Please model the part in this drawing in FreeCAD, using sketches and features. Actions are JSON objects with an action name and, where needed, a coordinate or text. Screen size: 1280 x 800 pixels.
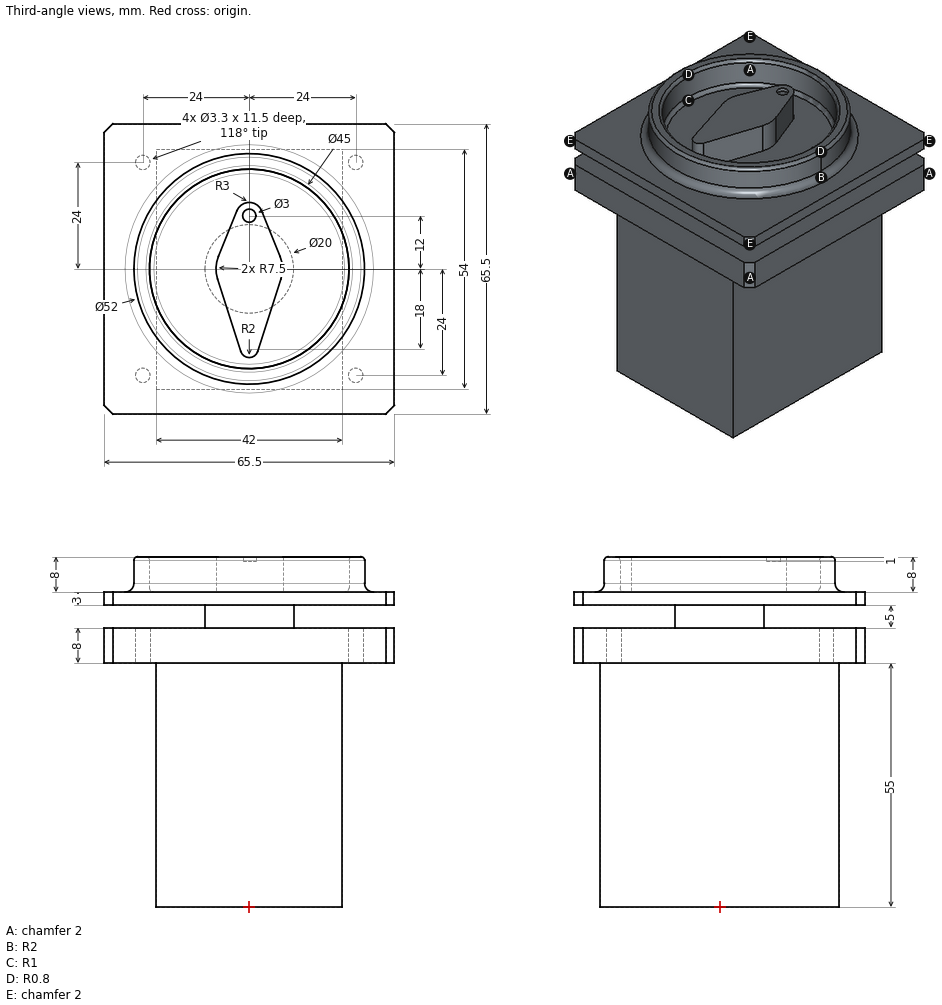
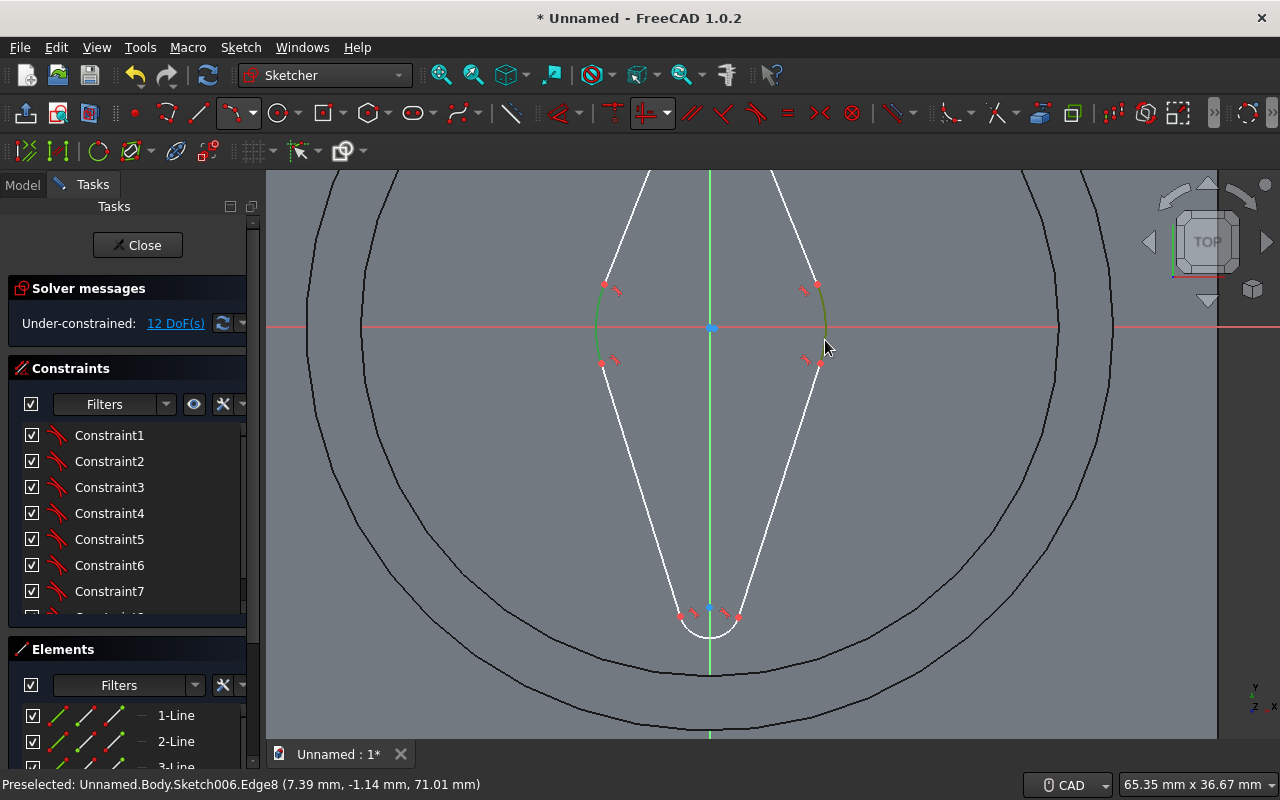
{"action": "left_click", "coordinate": [614, 114]}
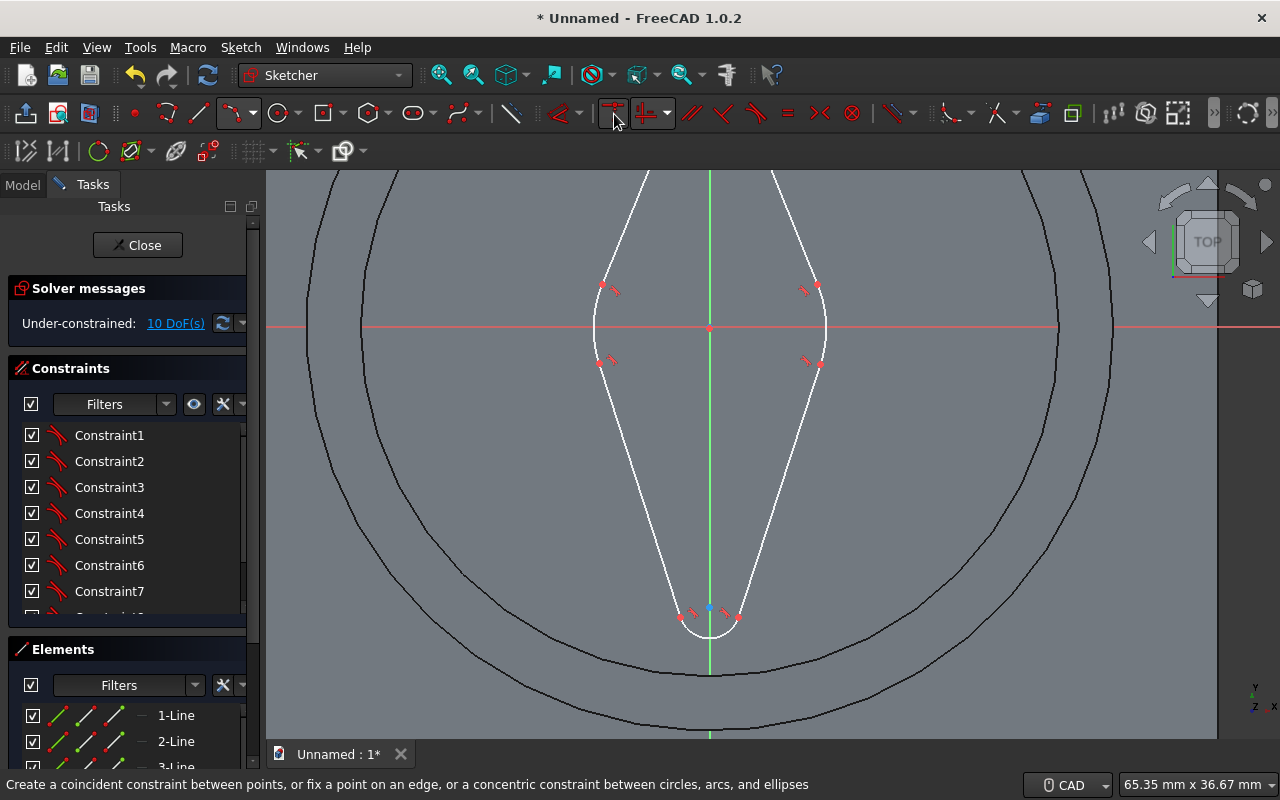
{"action": "scroll", "coordinate": [710, 328], "scroll_direction": "up", "scroll_amount": 2}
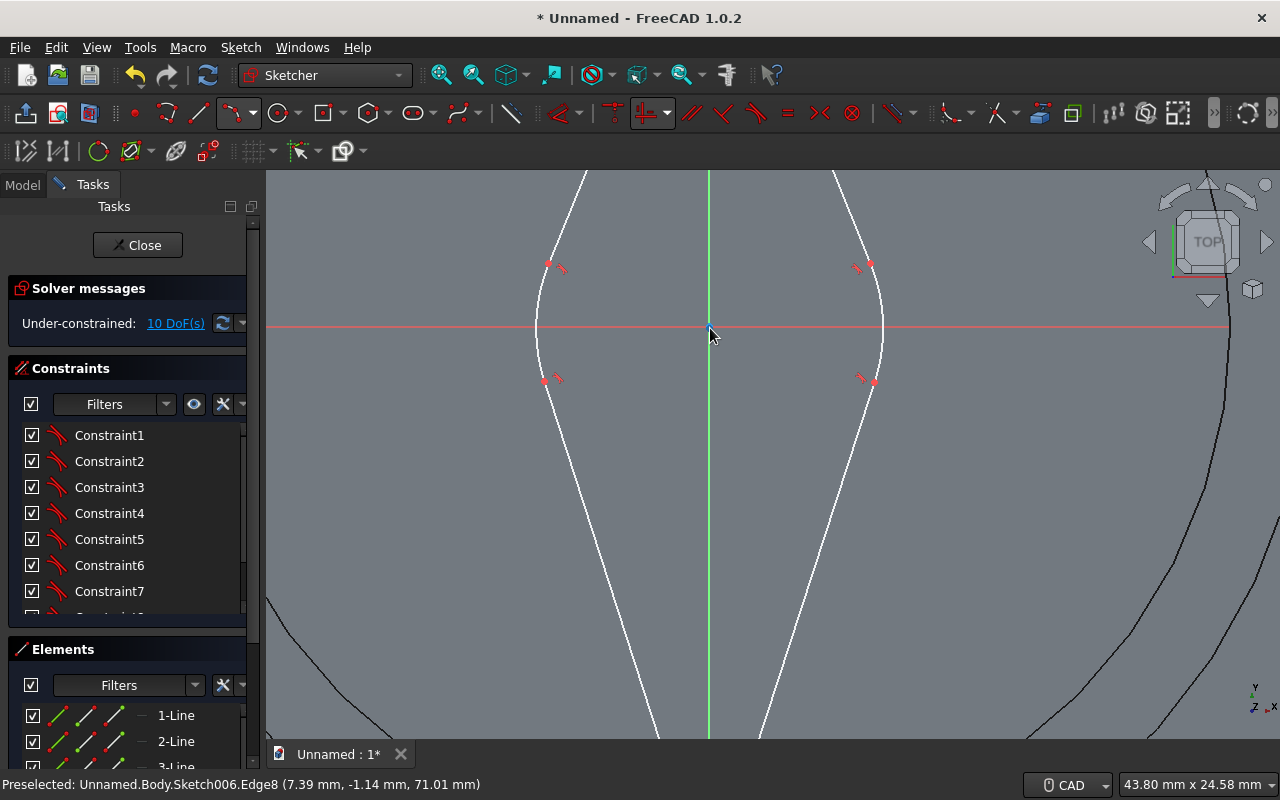
{"action": "left_click_drag", "start_coordinate": [699, 317], "coordinate": [719, 339]}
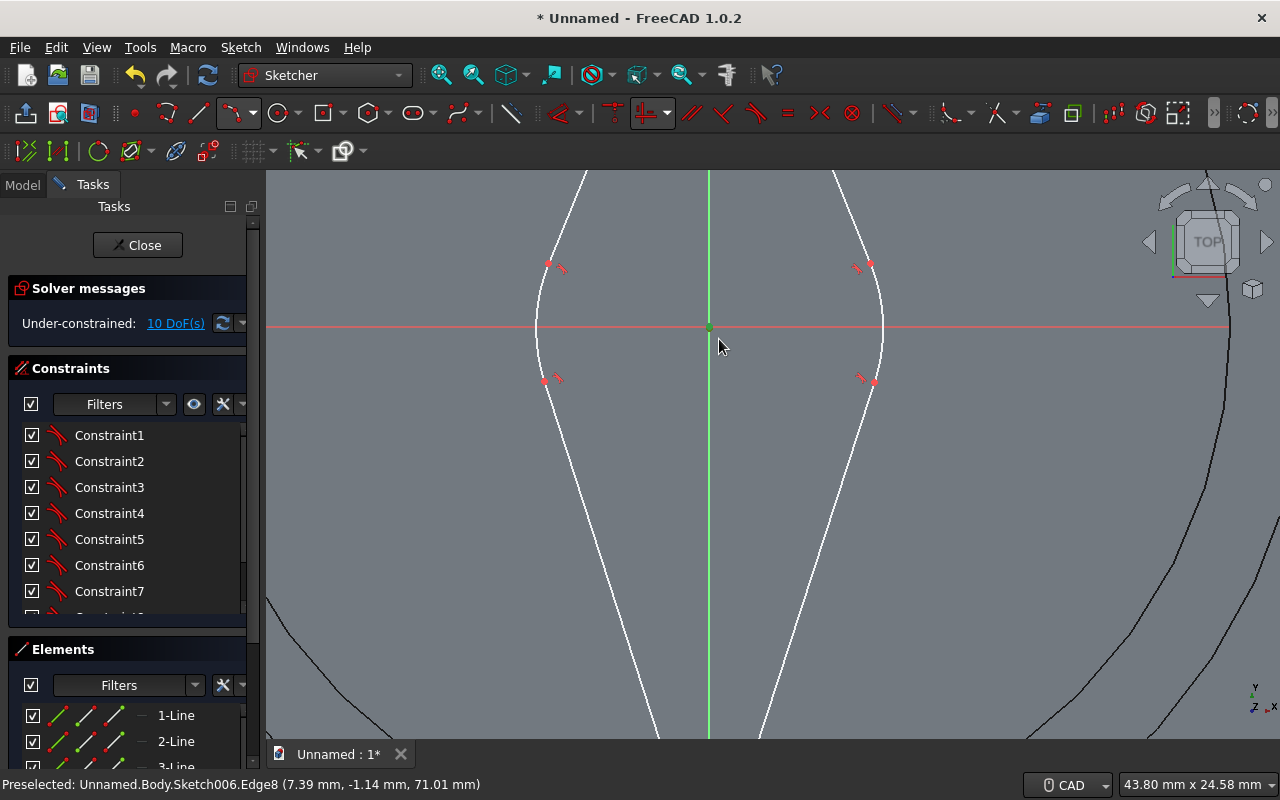
{"action": "left_click", "coordinate": [614, 114]}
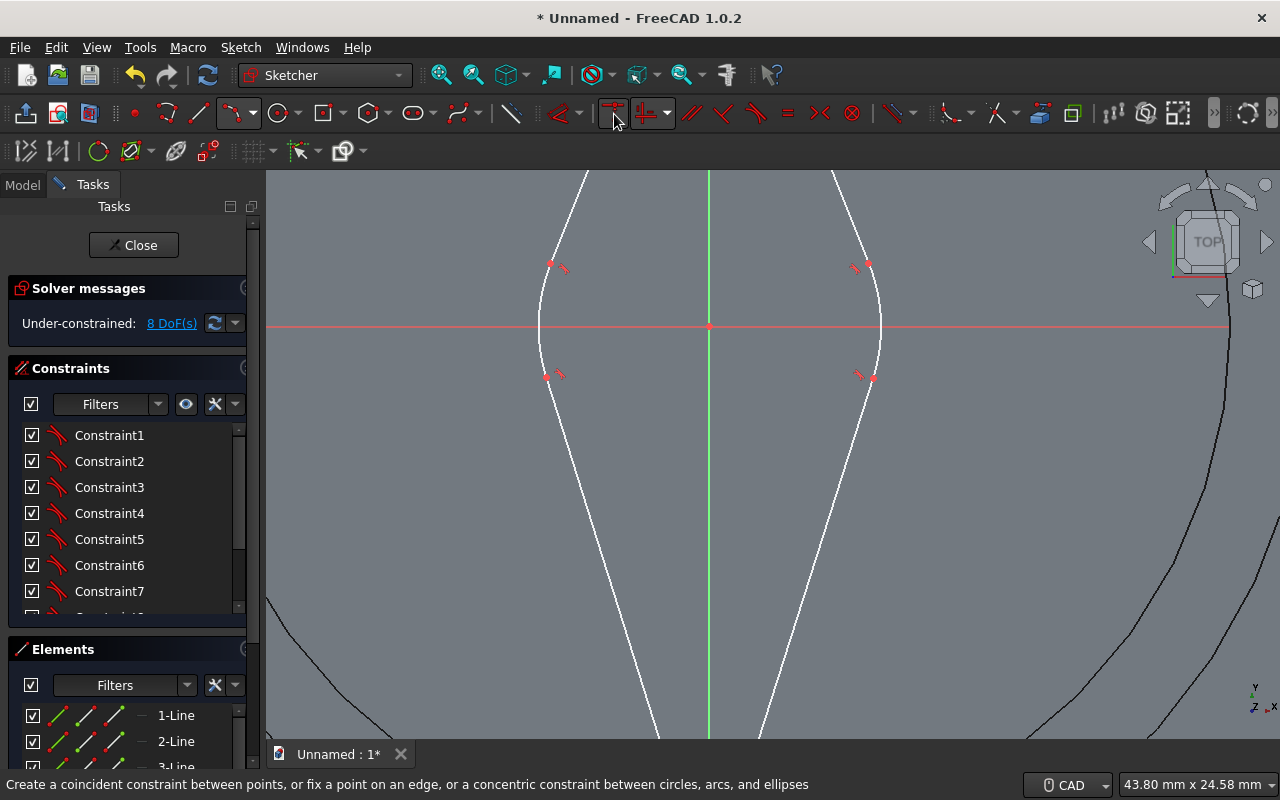
{"action": "left_click", "coordinate": [541, 297]}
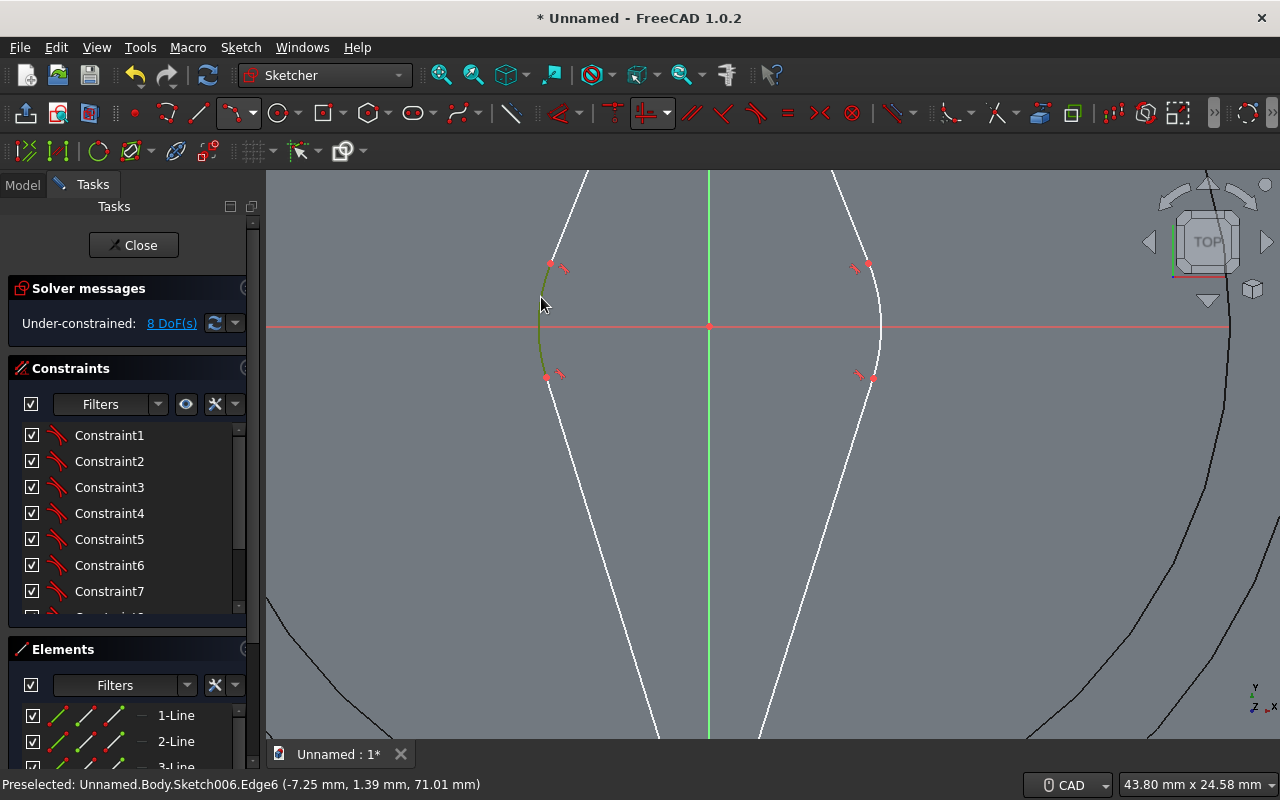
{"action": "left_click", "coordinate": [880, 344]}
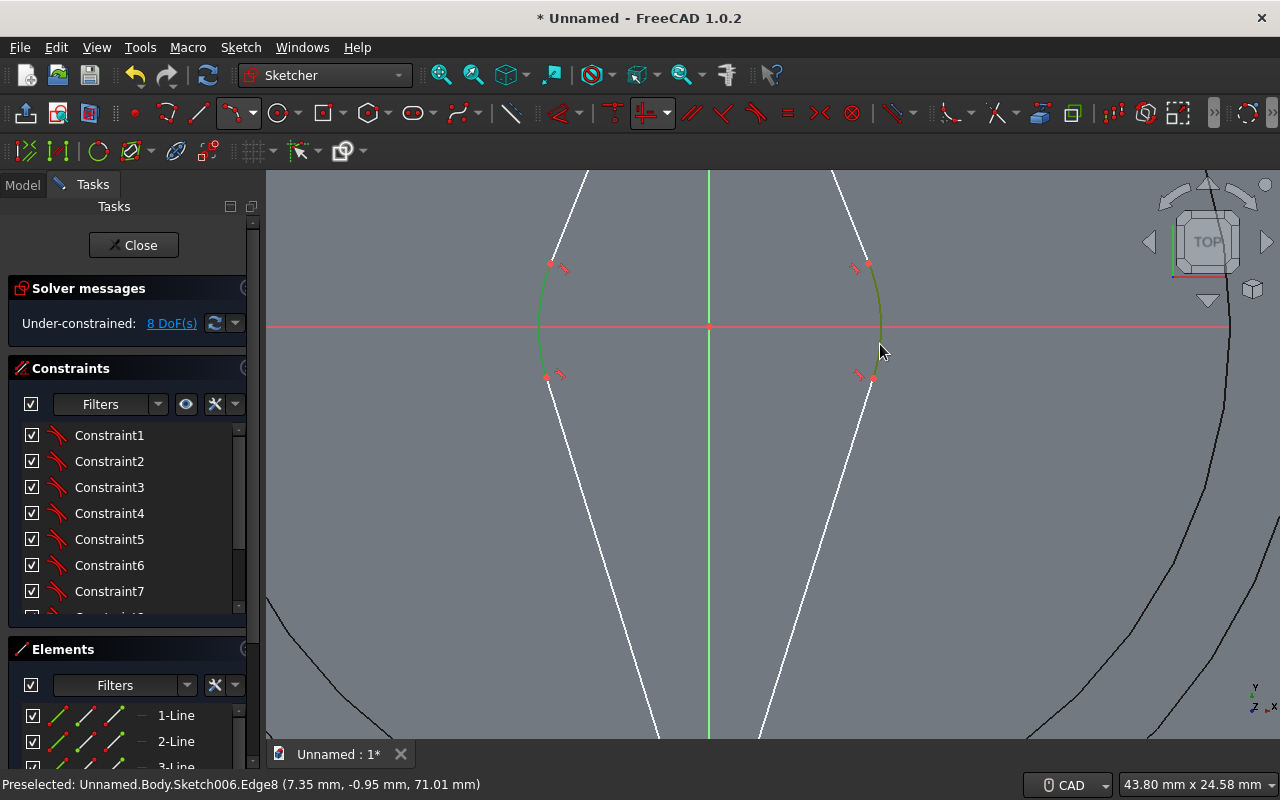
{"action": "left_click", "coordinate": [788, 114]}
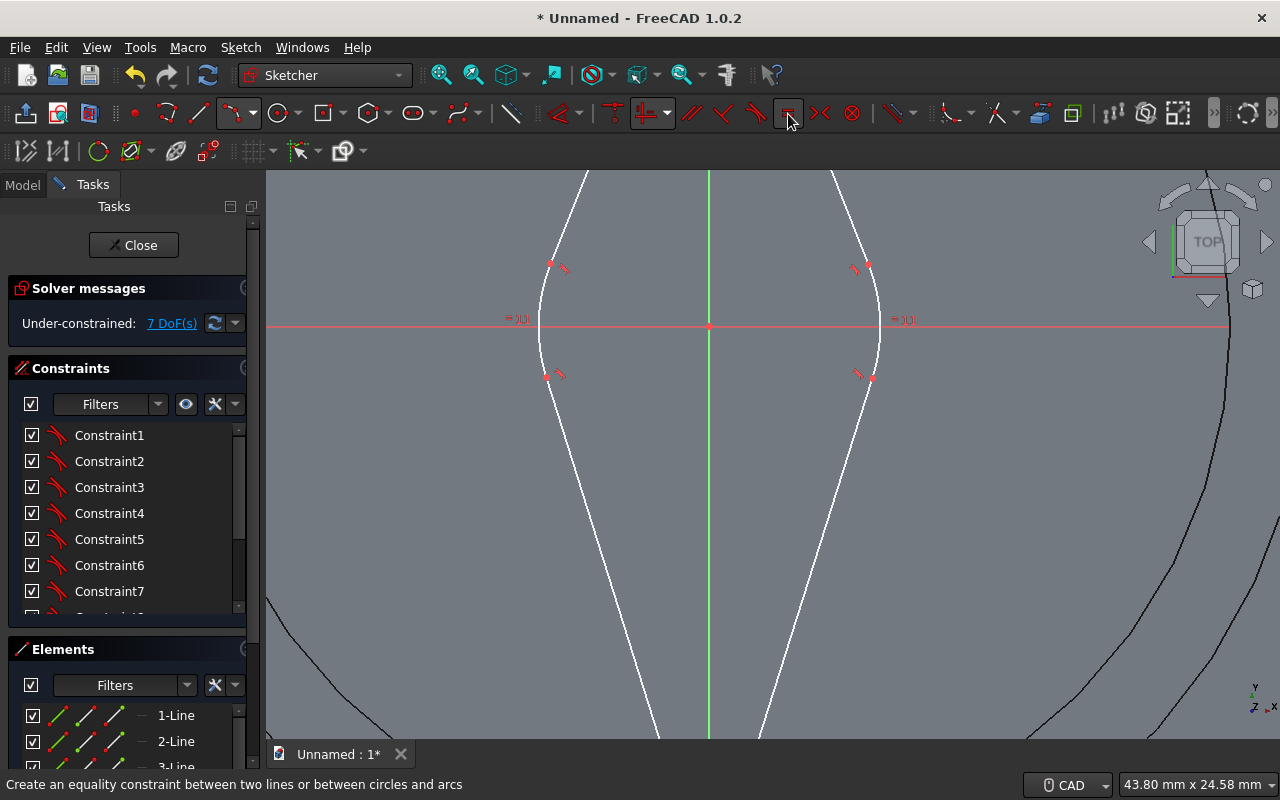
{"action": "scroll", "coordinate": [700, 511], "scroll_direction": "down", "scroll_amount": 4}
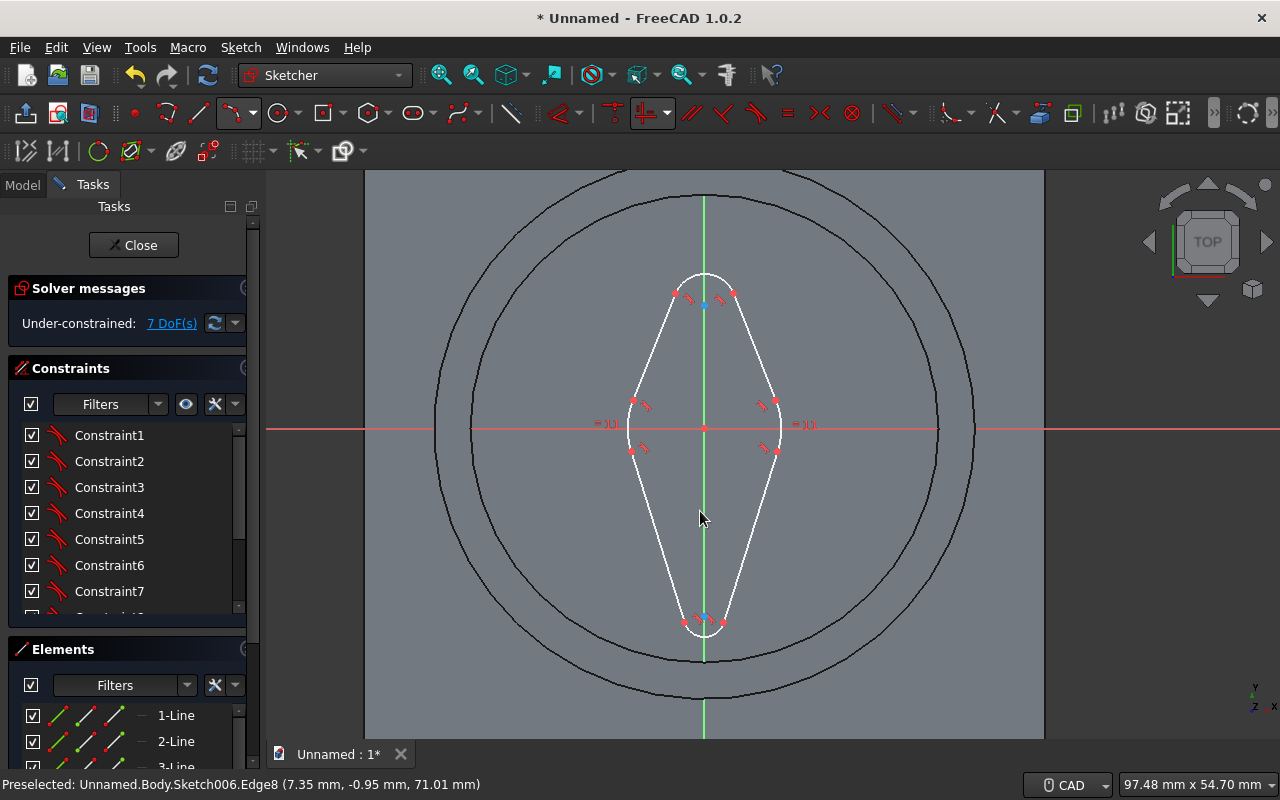
{"action": "left_click", "coordinate": [705, 305]}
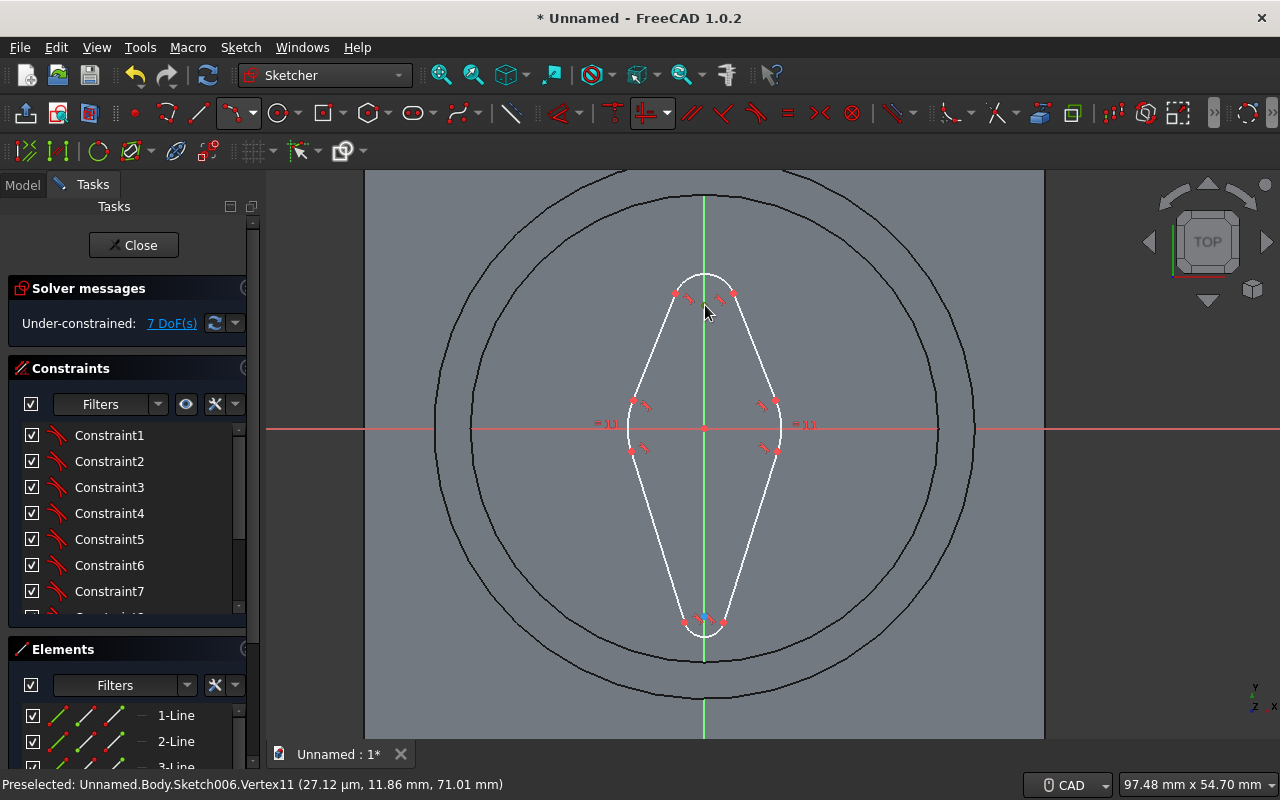
{"action": "left_click", "coordinate": [704, 674]}